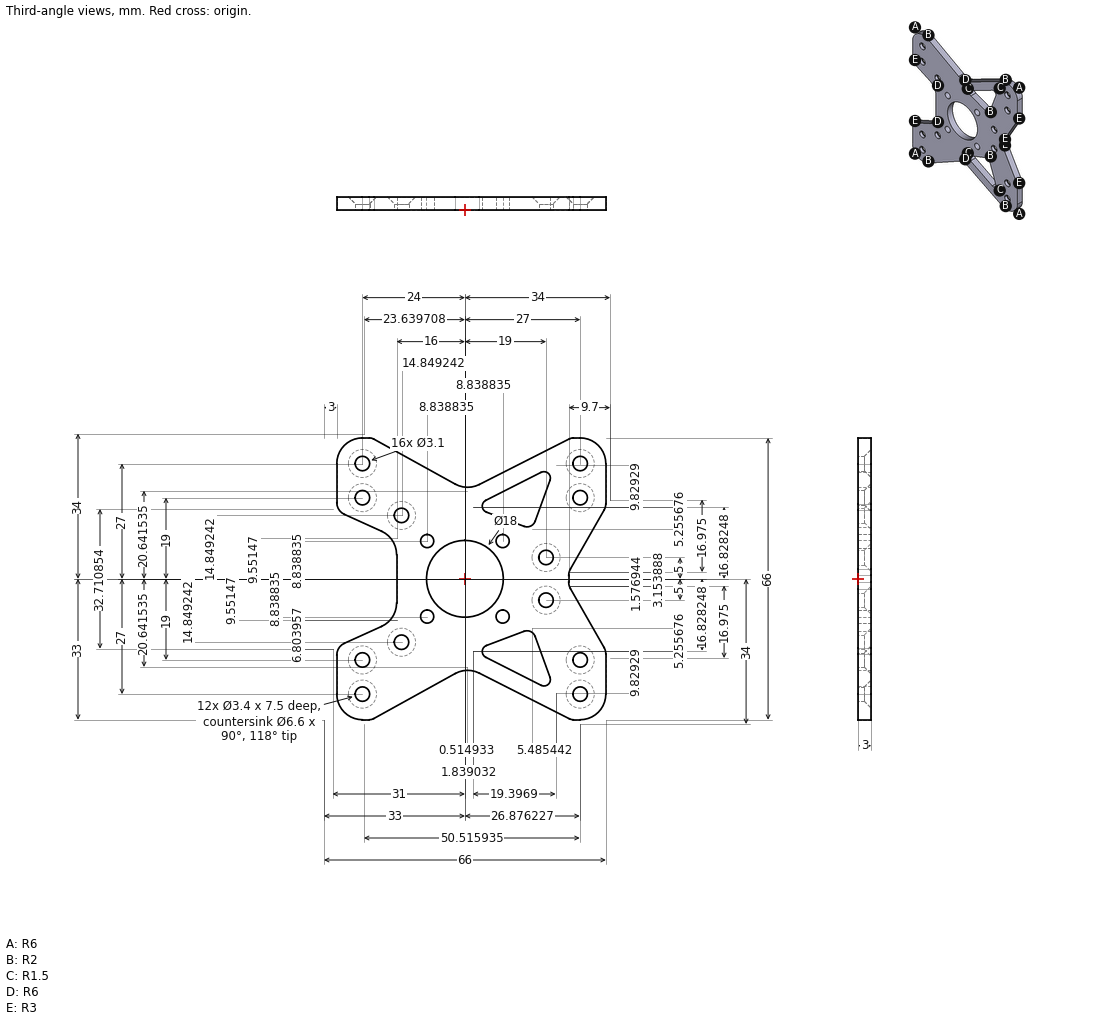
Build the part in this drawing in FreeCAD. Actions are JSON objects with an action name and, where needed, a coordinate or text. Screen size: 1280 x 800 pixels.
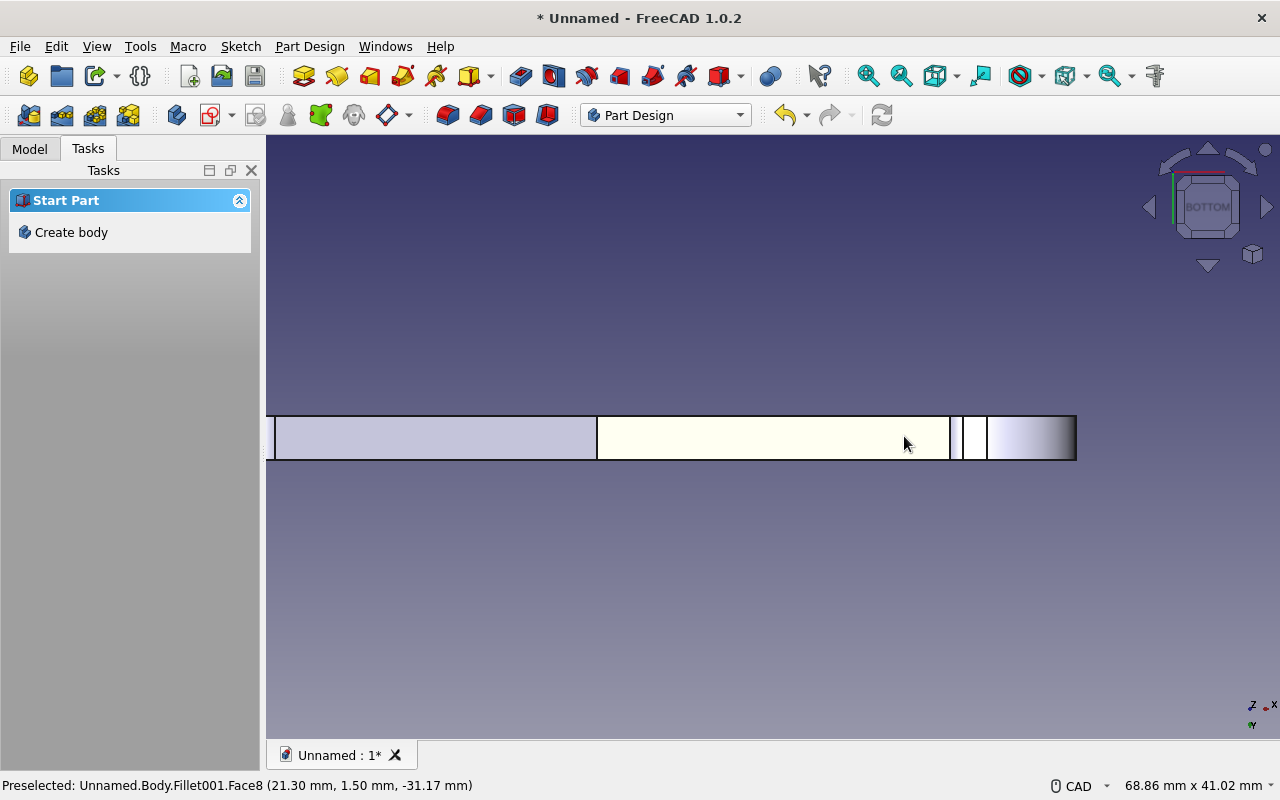
{"action": "key", "text": "v f"}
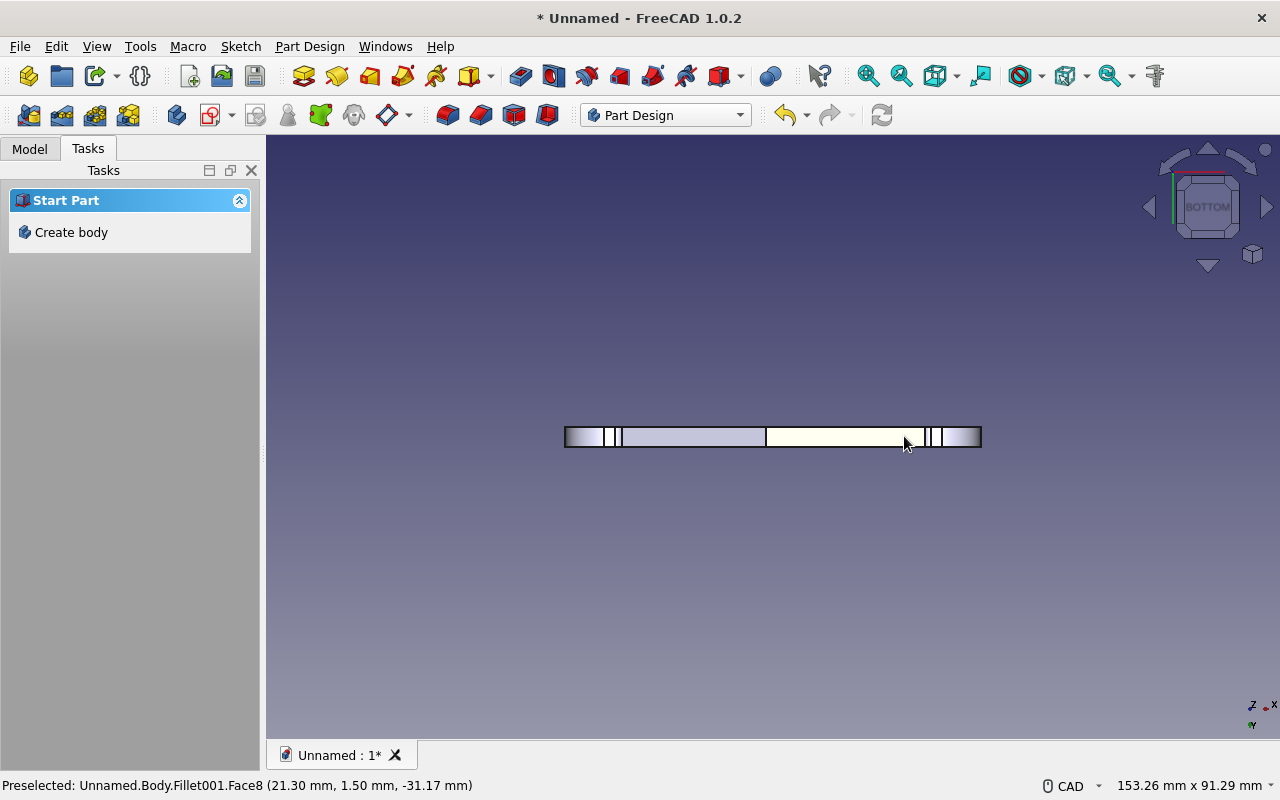
{"action": "key", "text": "4"}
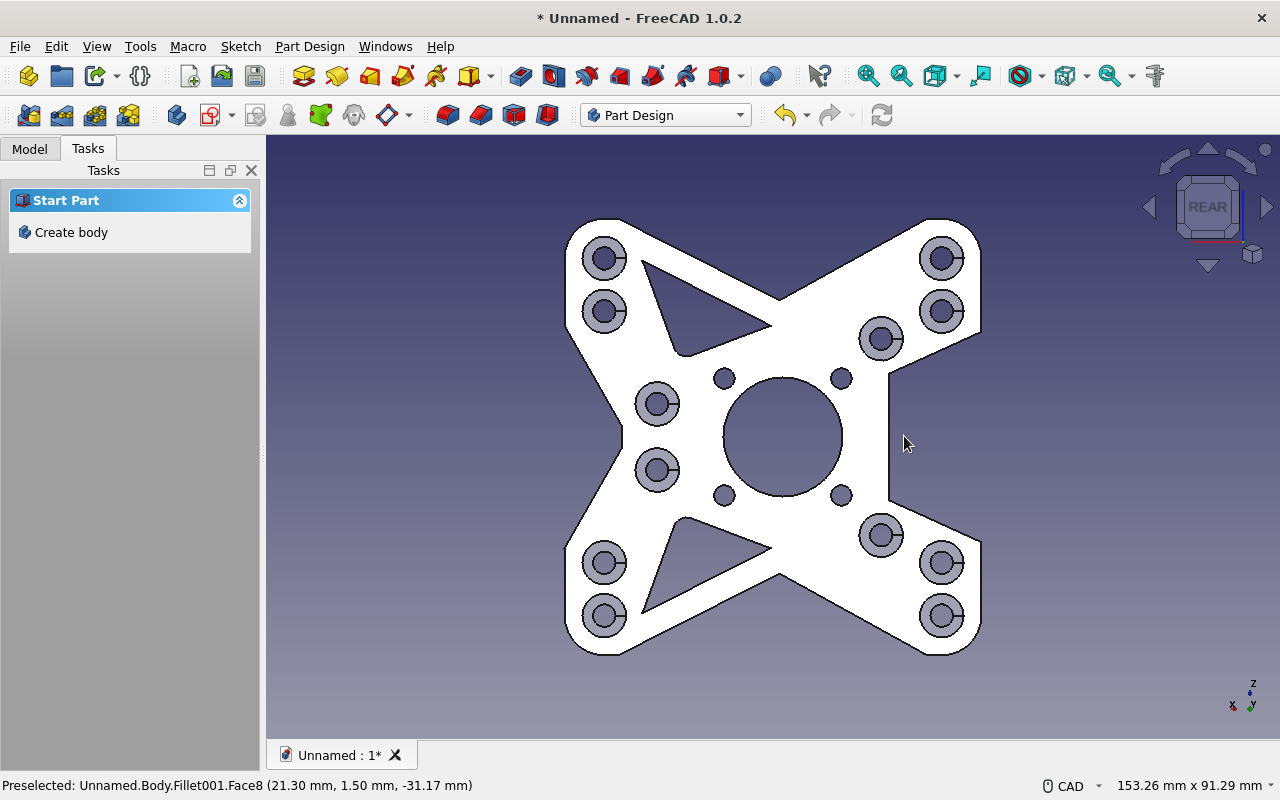
{"action": "scroll", "coordinate": [642, 260], "scroll_direction": "up", "scroll_amount": 4}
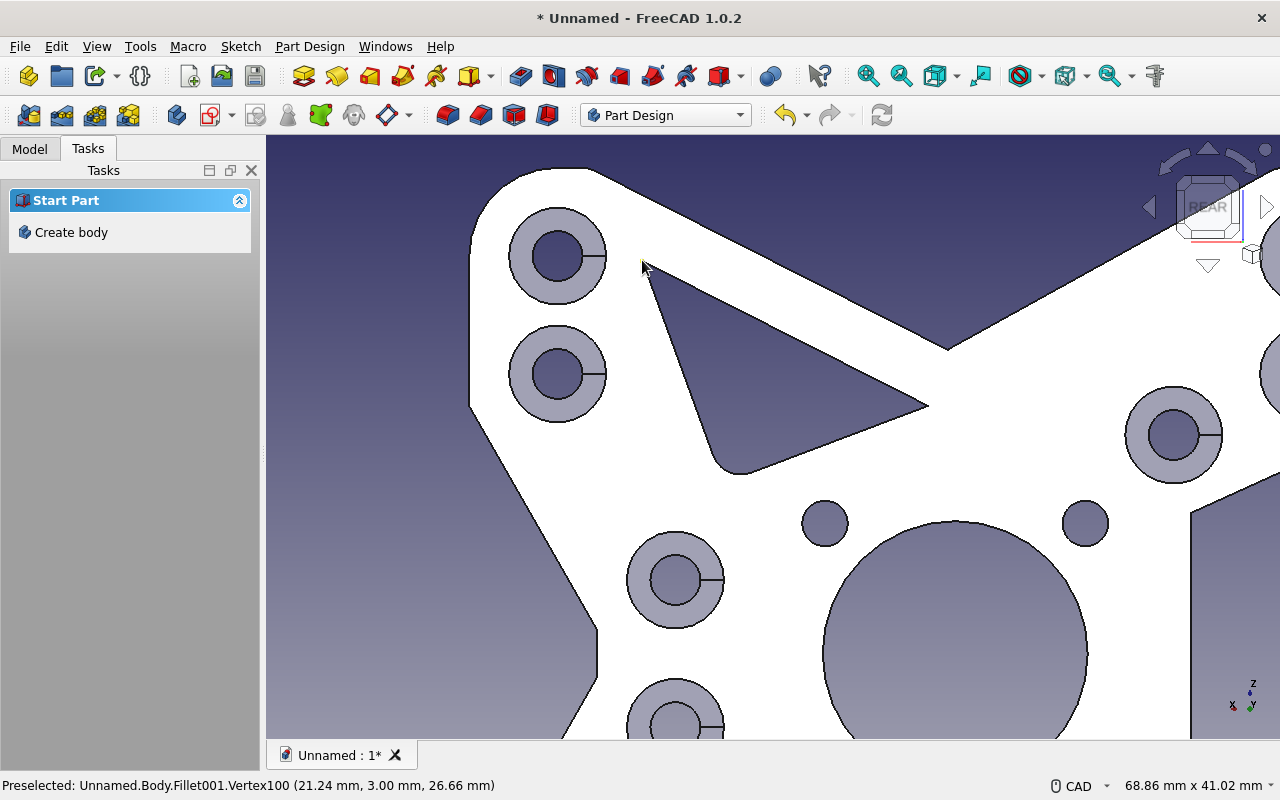
{"action": "left_click", "coordinate": [869, 76]}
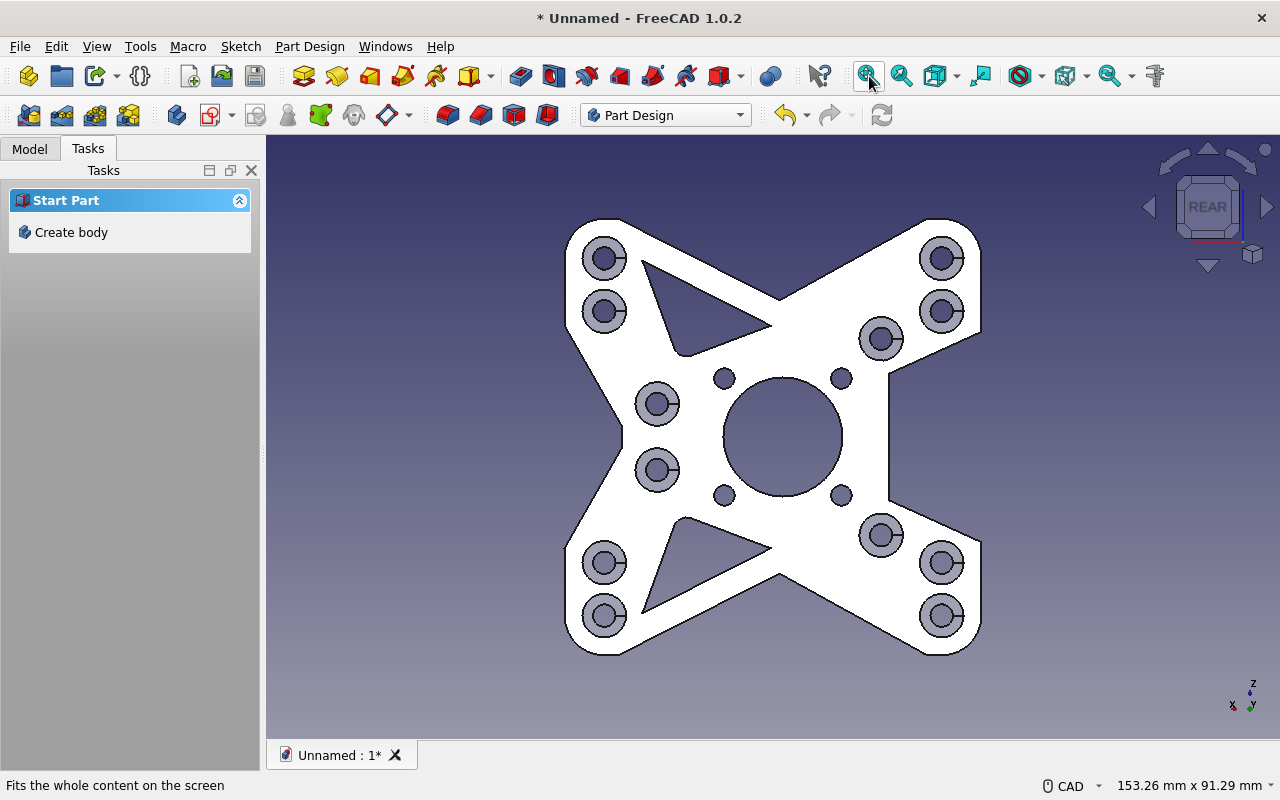
{"action": "key", "text": "6"}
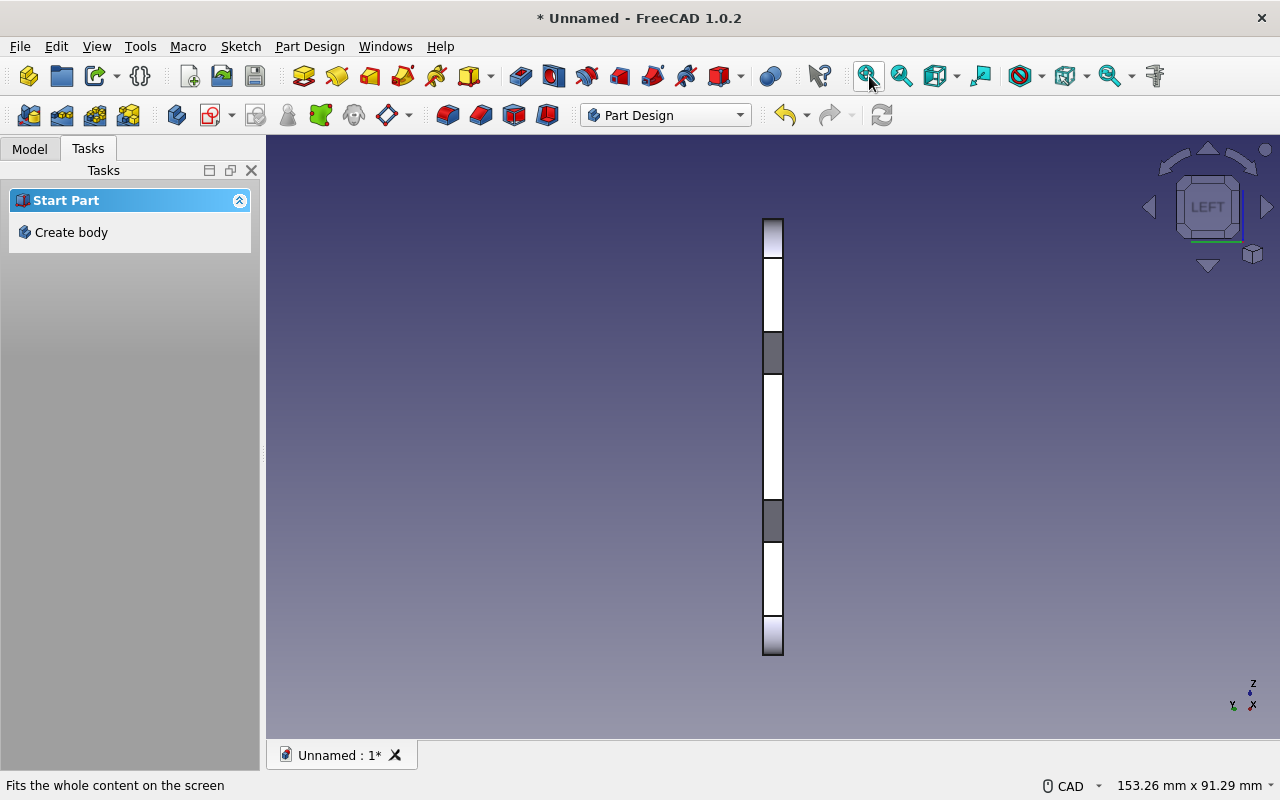
{"action": "scroll", "coordinate": [773, 260], "scroll_direction": "up", "scroll_amount": 4}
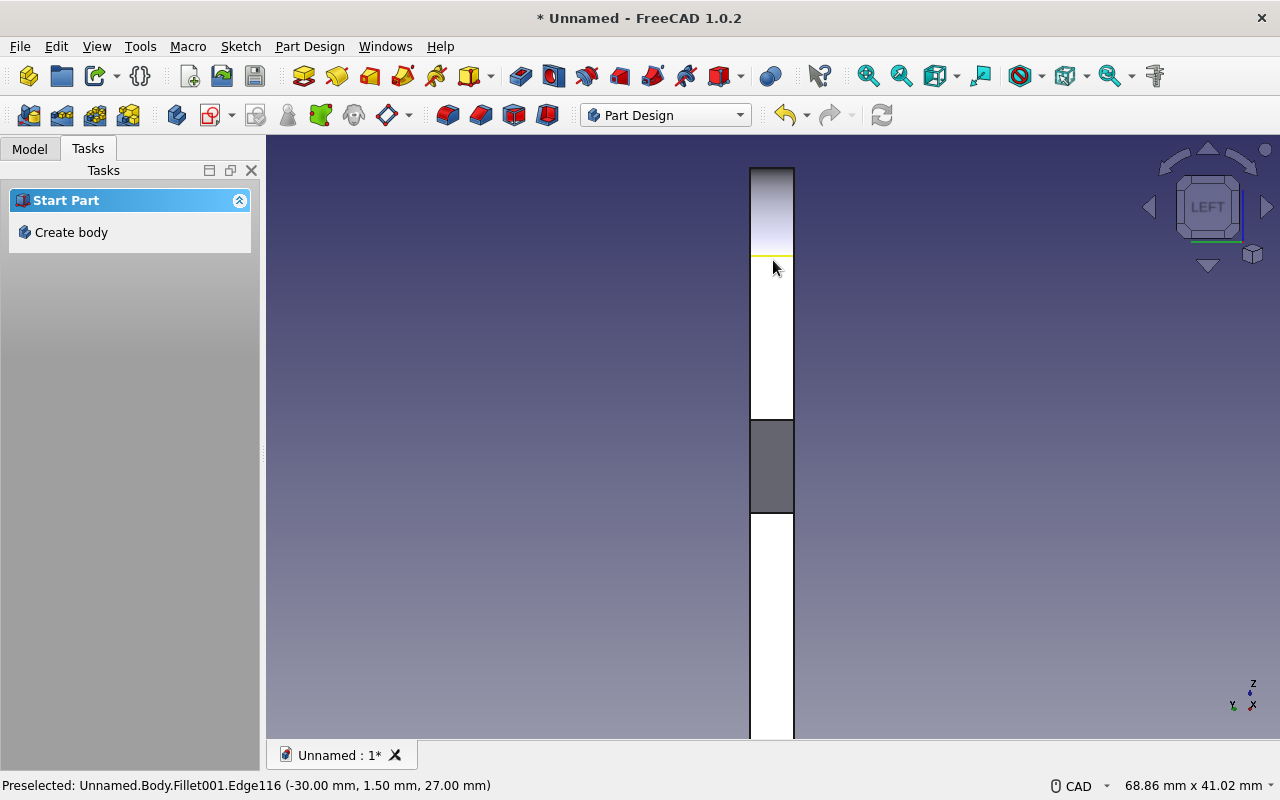
{"action": "left_click", "coordinate": [869, 76]}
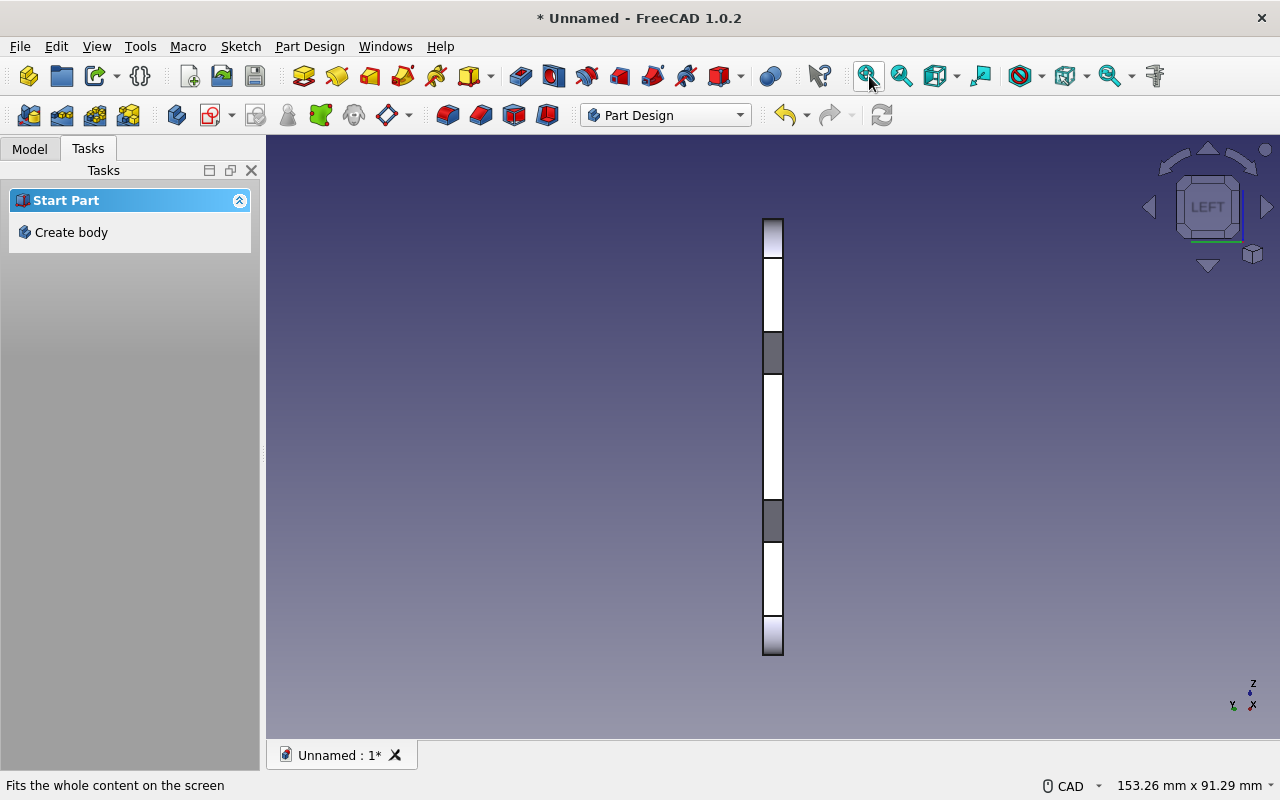
{"action": "key", "text": "v 3"}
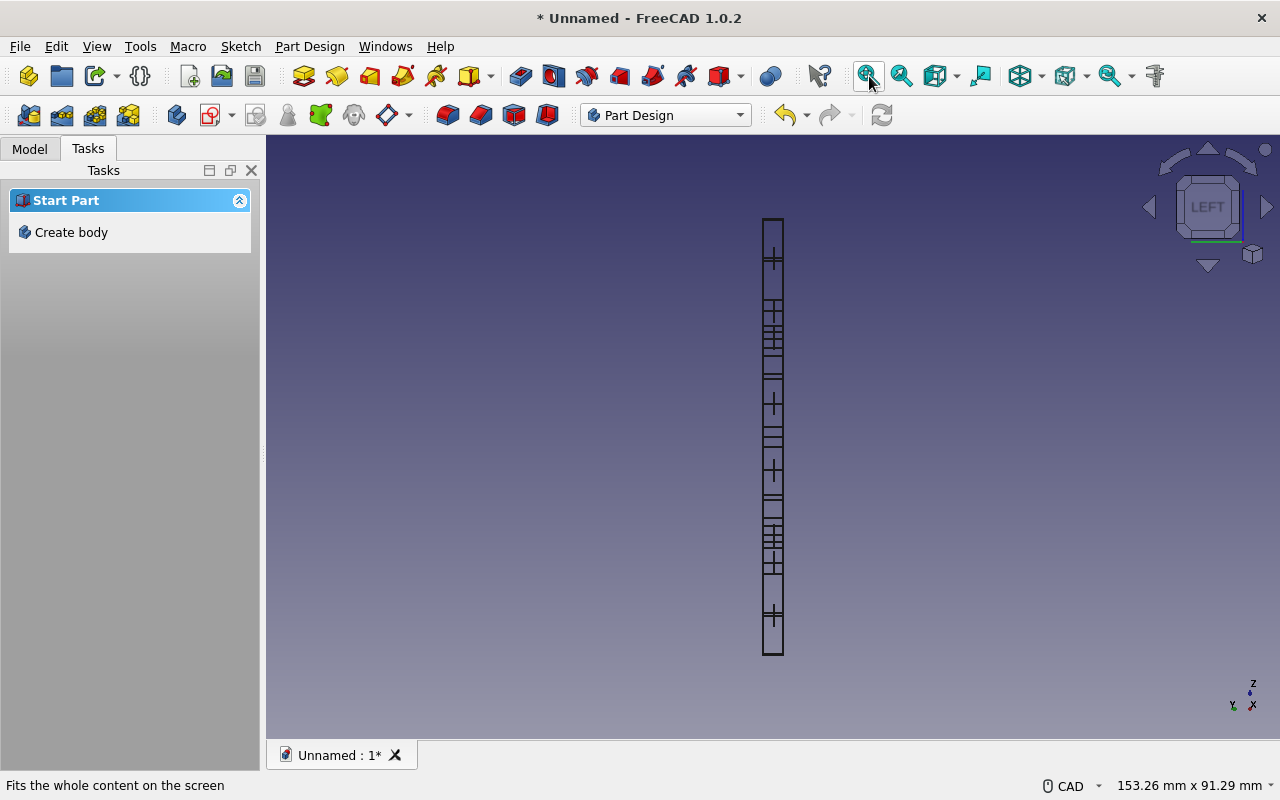
{"action": "key", "text": "0"}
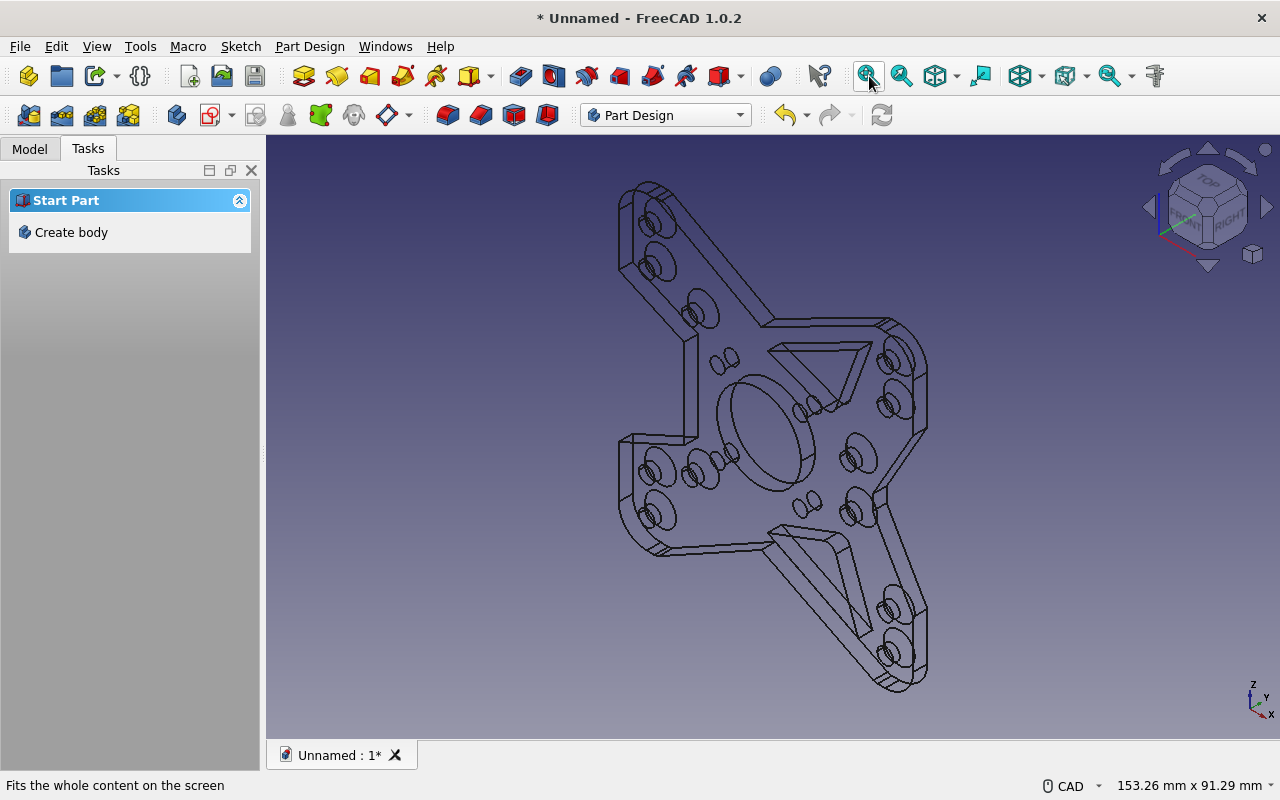
{"action": "left_click", "coordinate": [865, 345]}